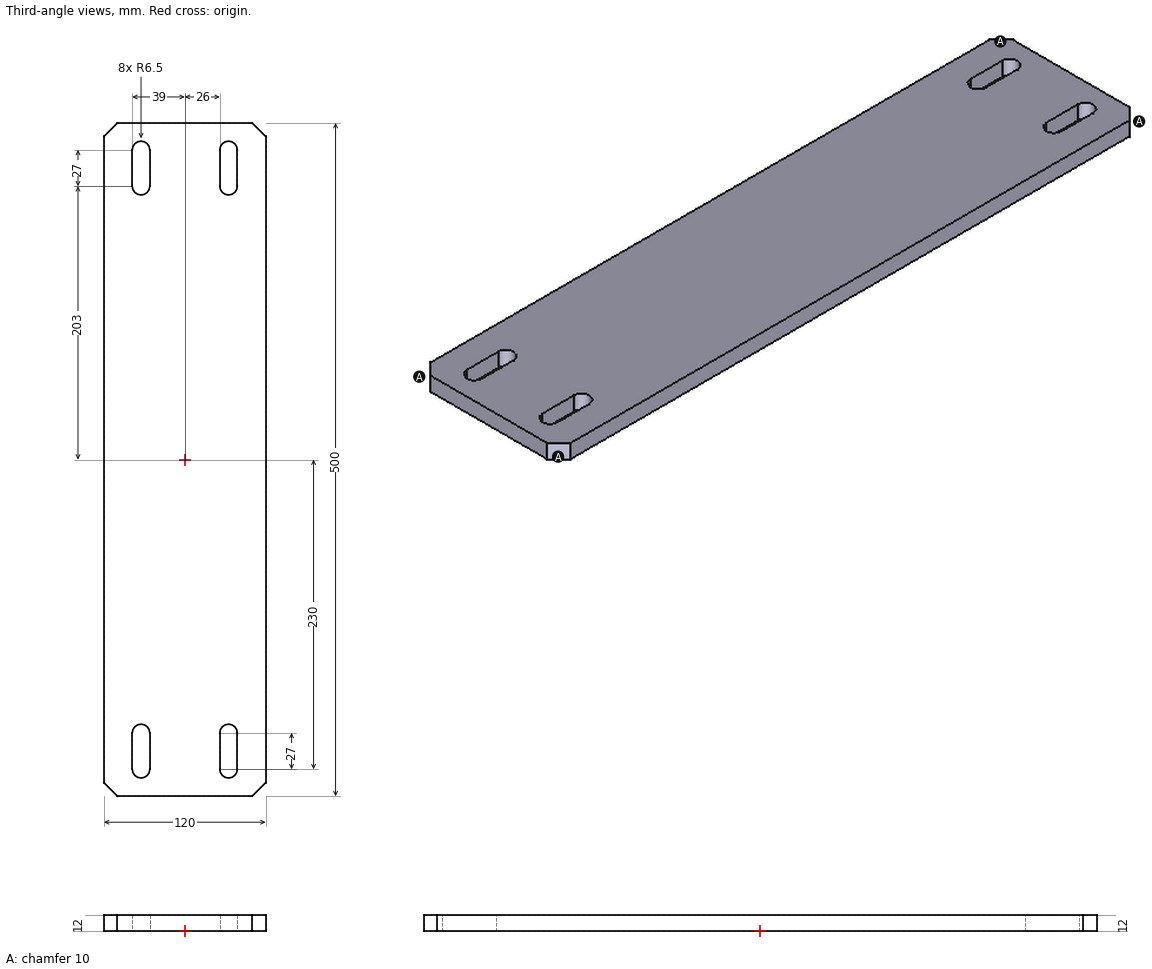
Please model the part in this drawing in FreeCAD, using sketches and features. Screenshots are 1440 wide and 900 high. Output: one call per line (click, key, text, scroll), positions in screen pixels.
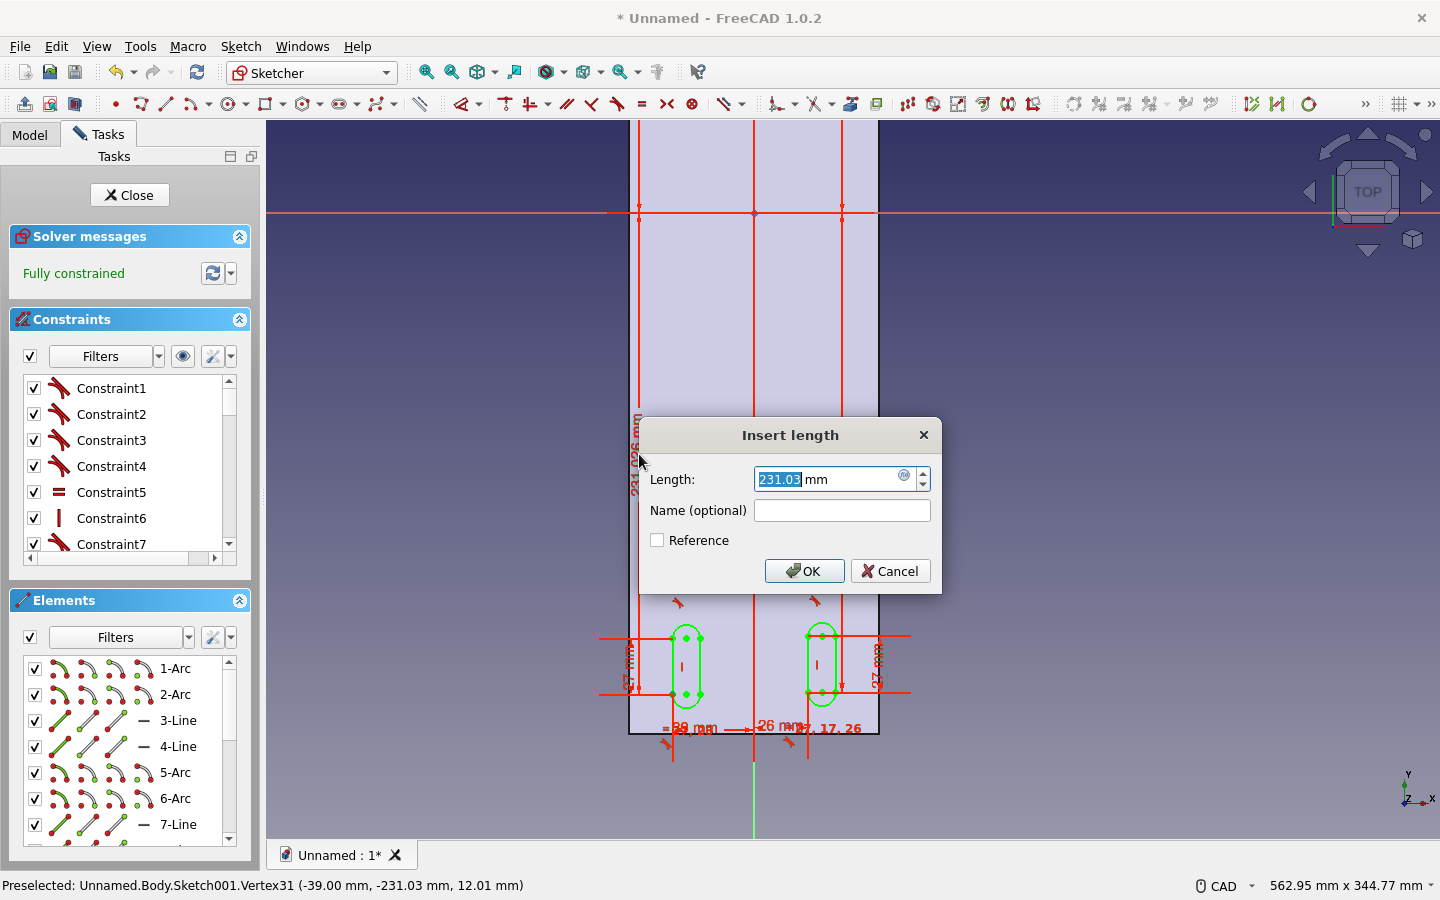
text(230)
key(Return)
key(Escape)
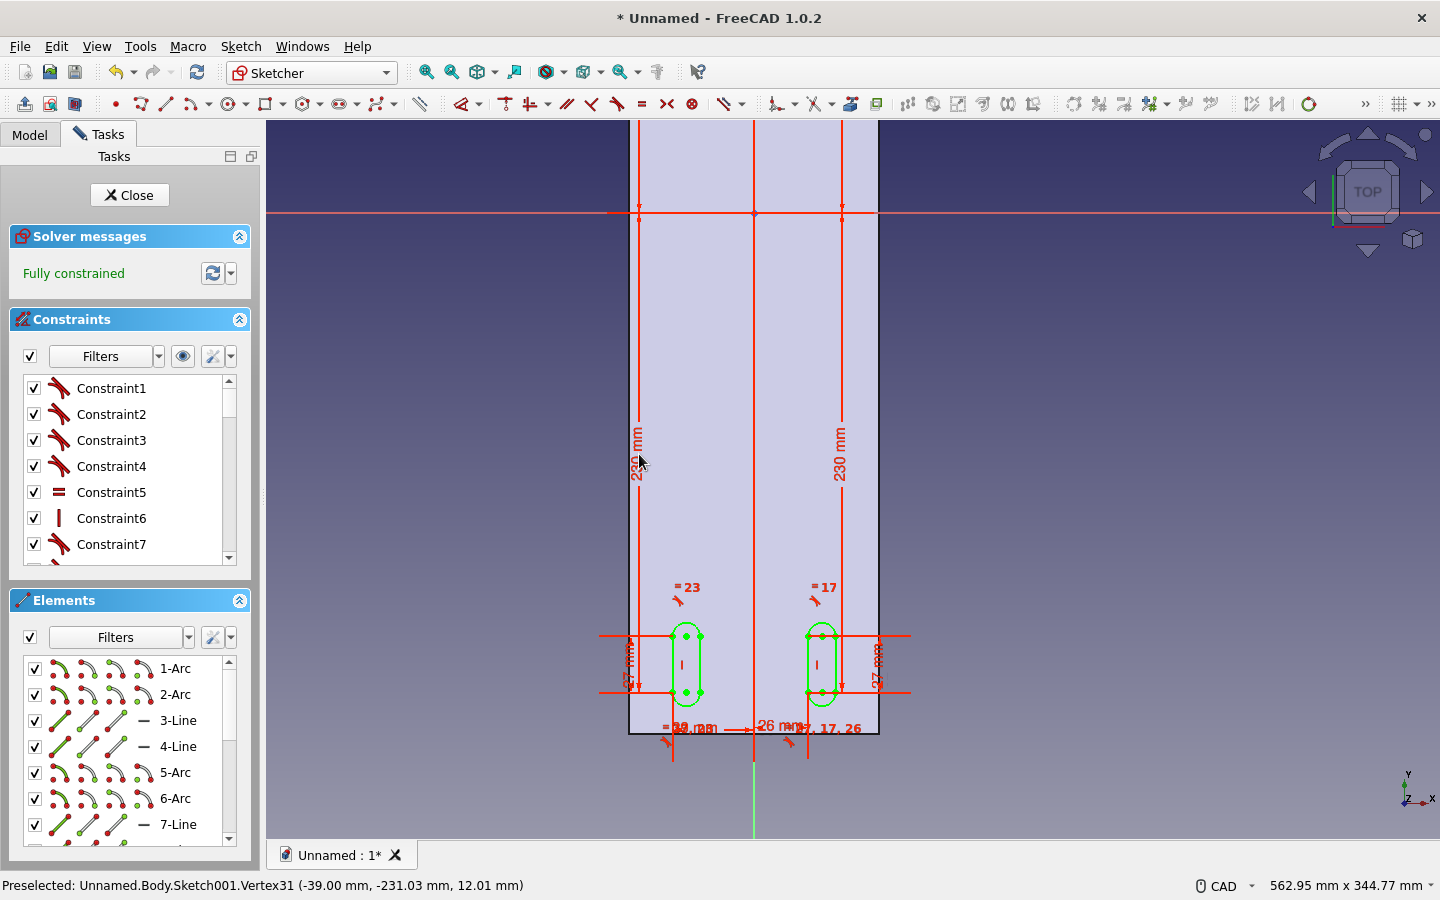
click(130, 195)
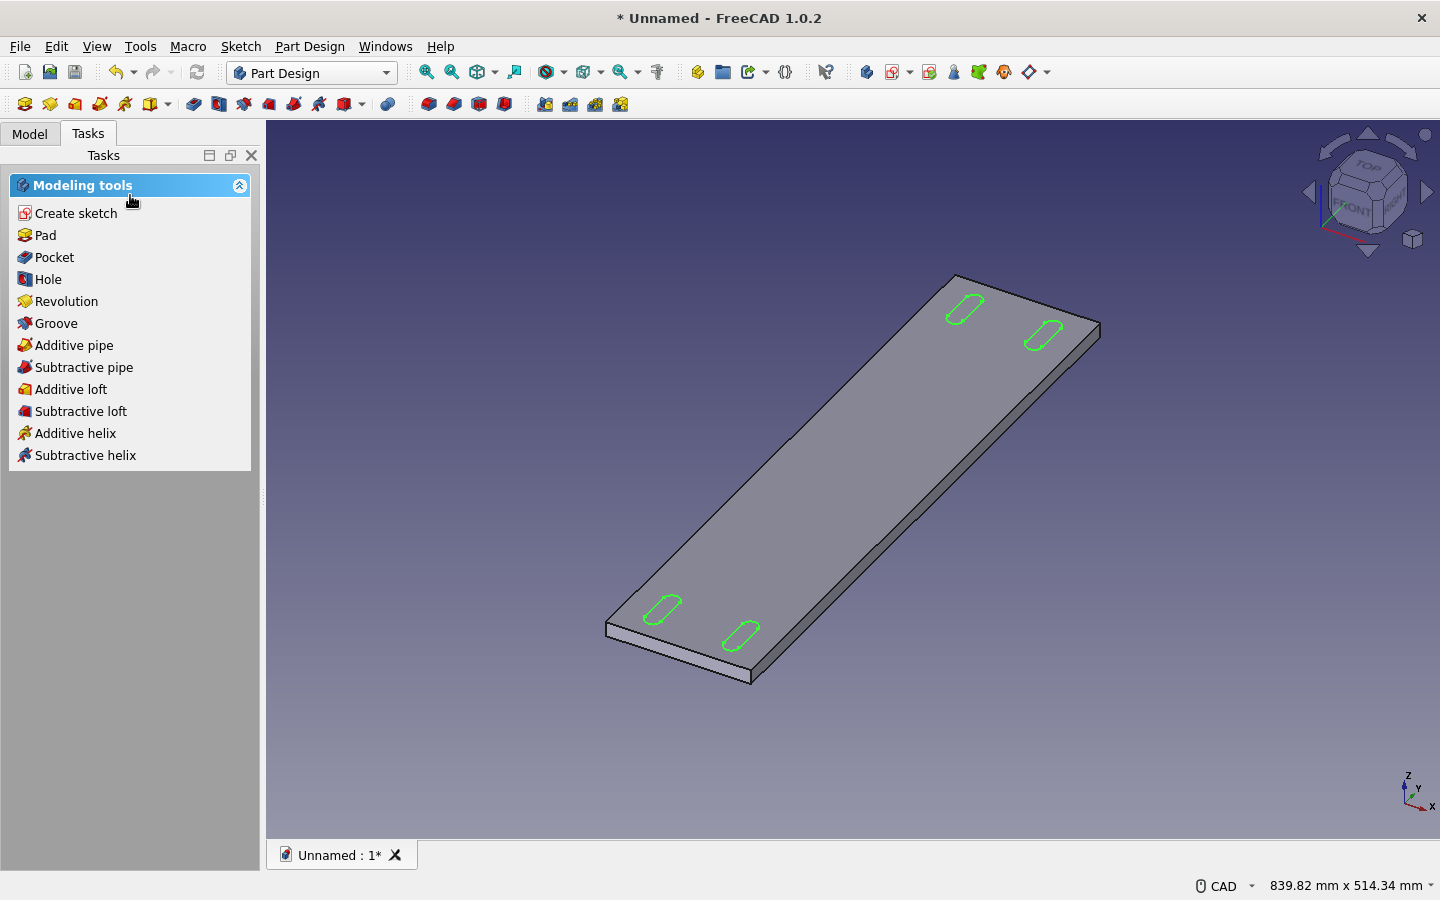
click(194, 104)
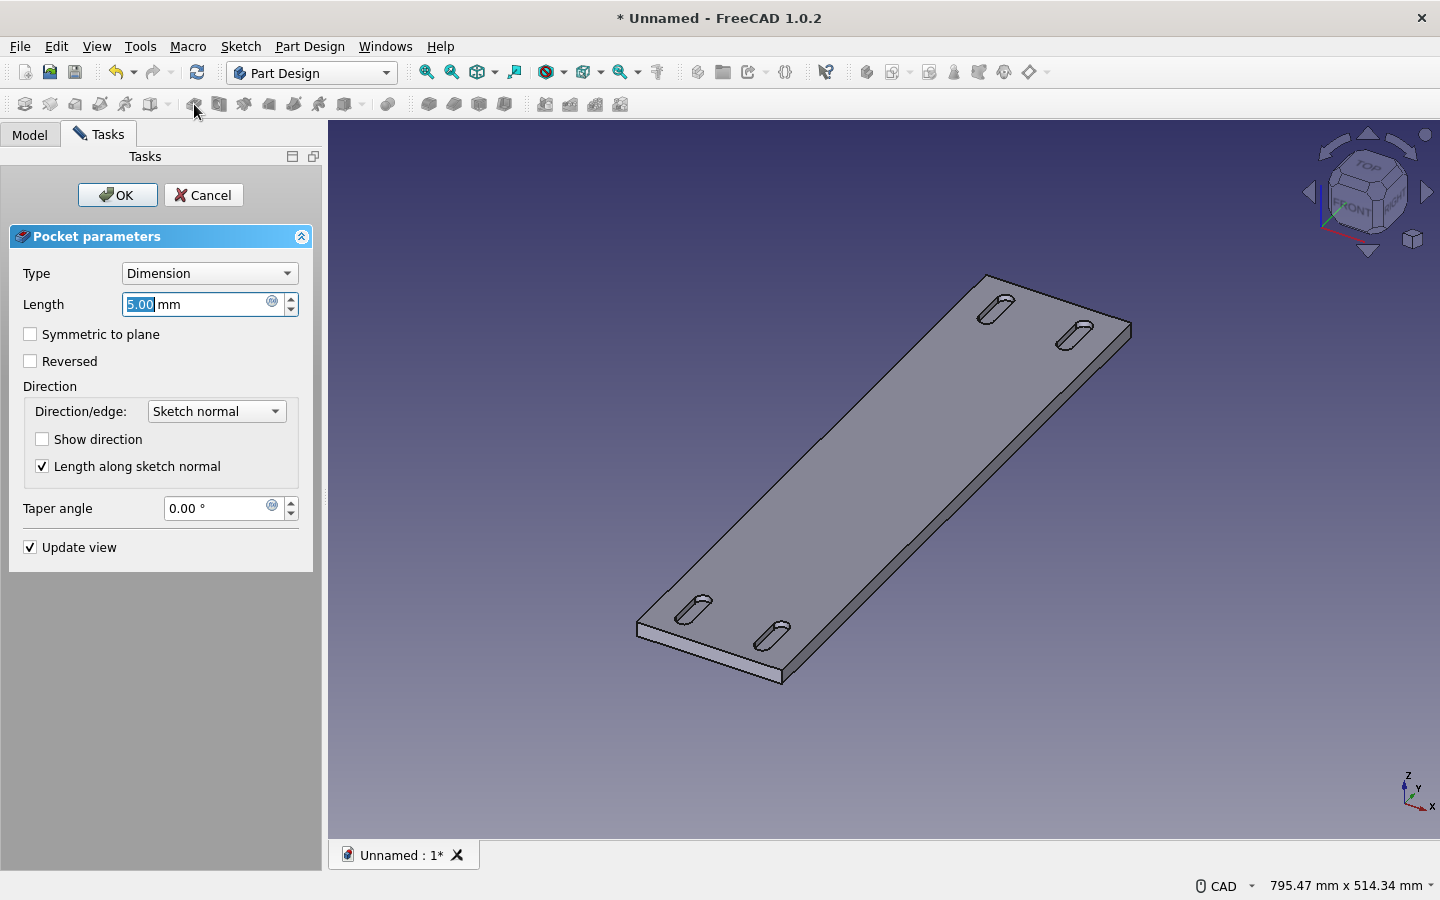
text(12)
key(Tab)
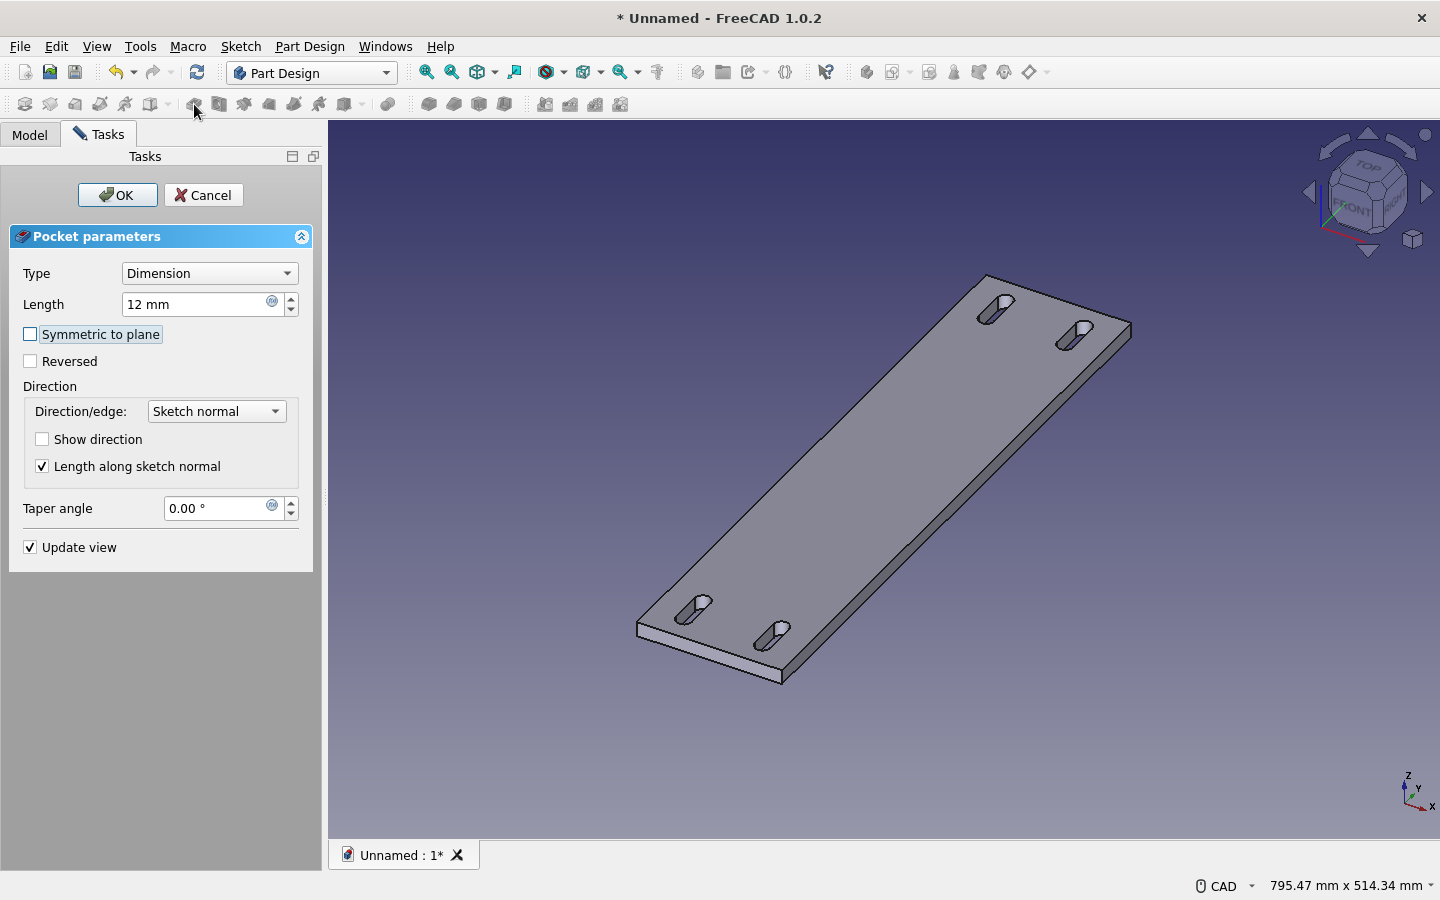
click(118, 195)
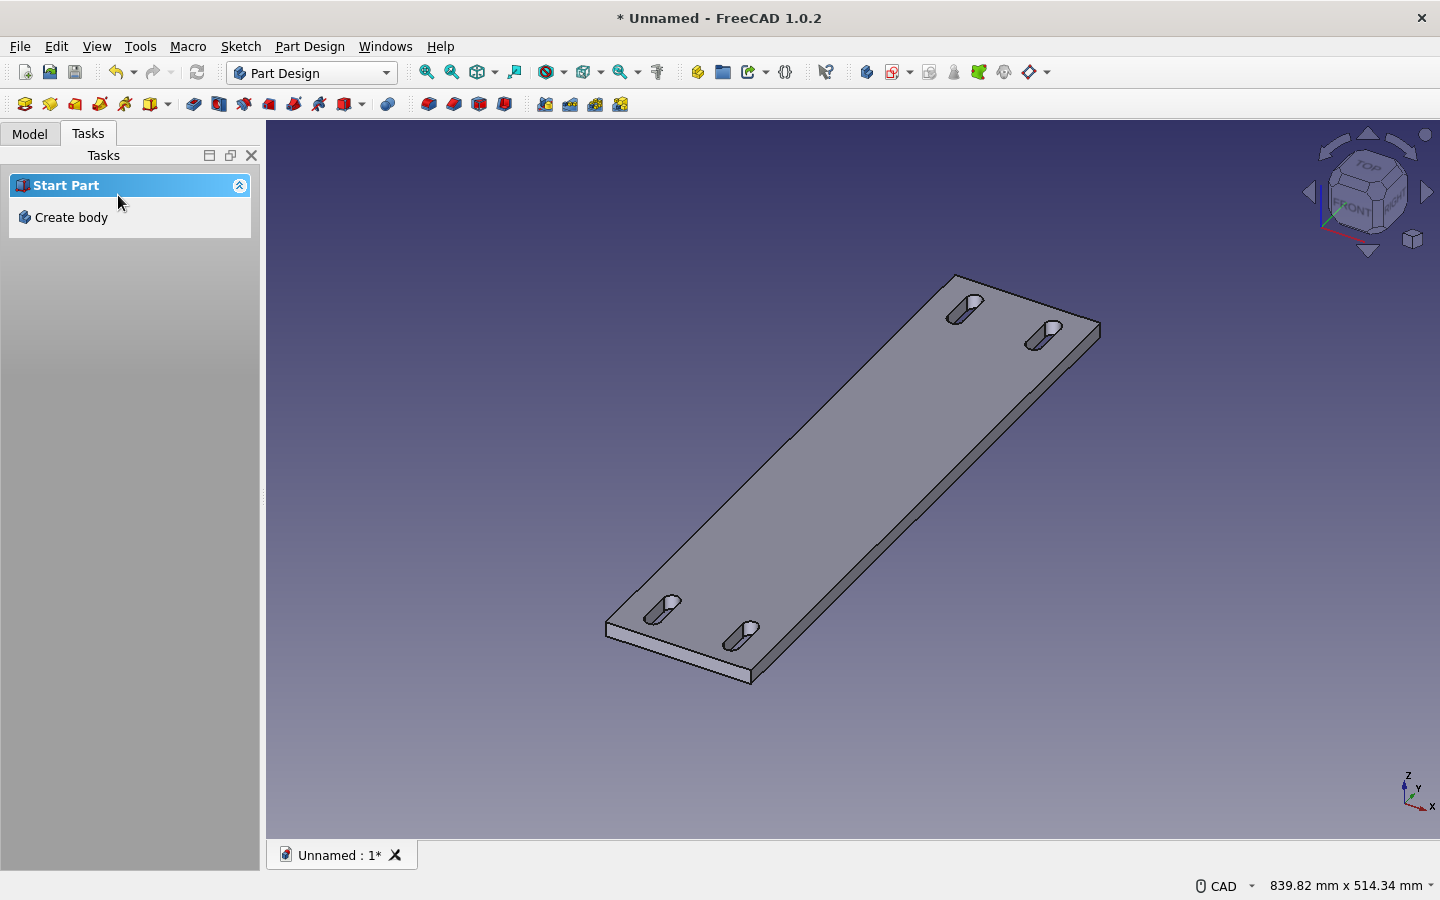
click(751, 676)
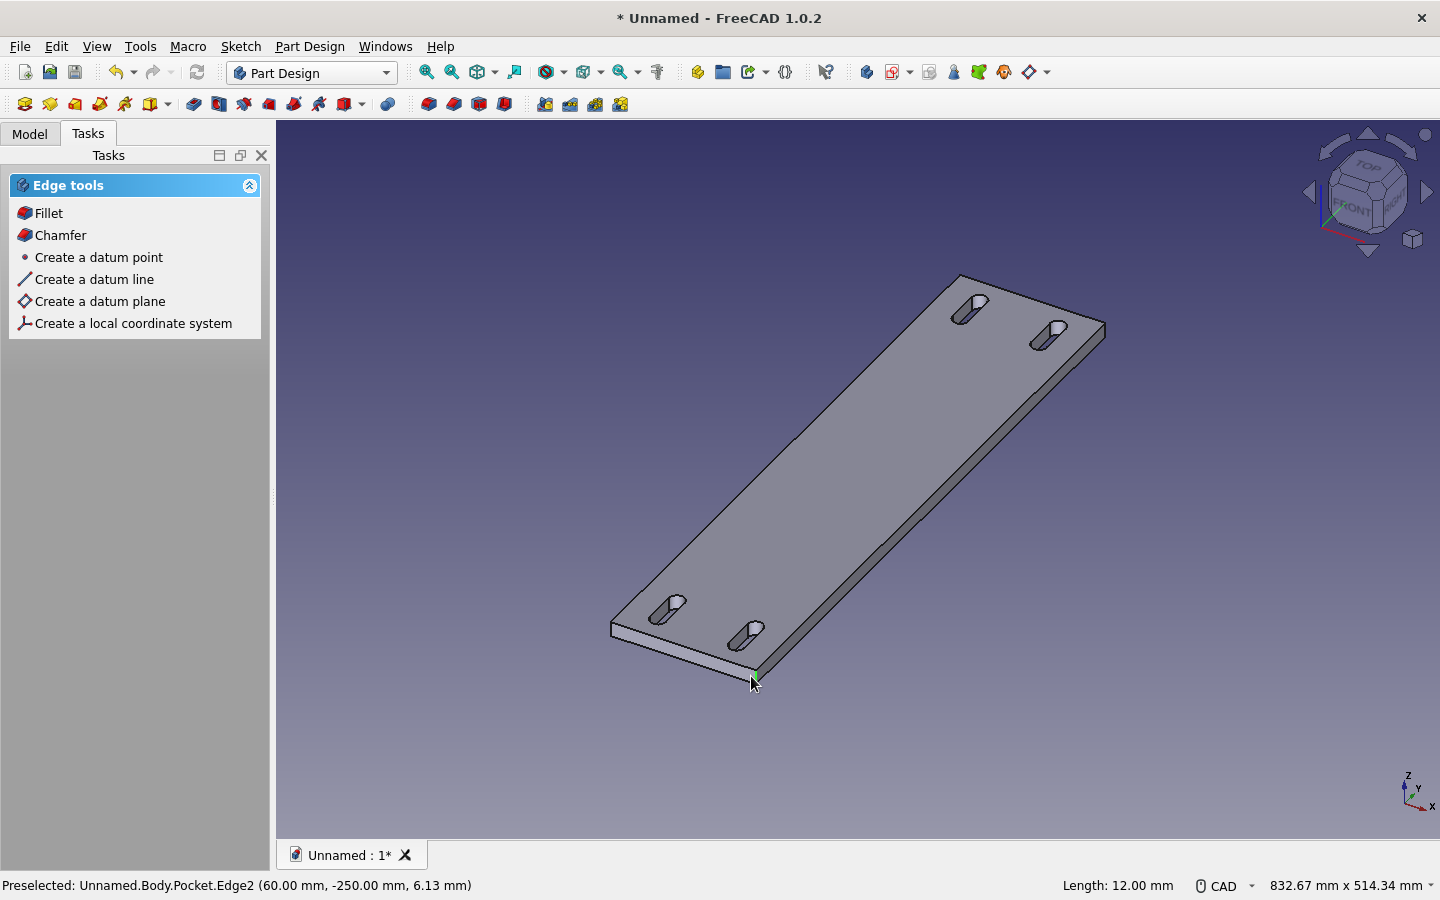
scroll(611, 628, up, 5)